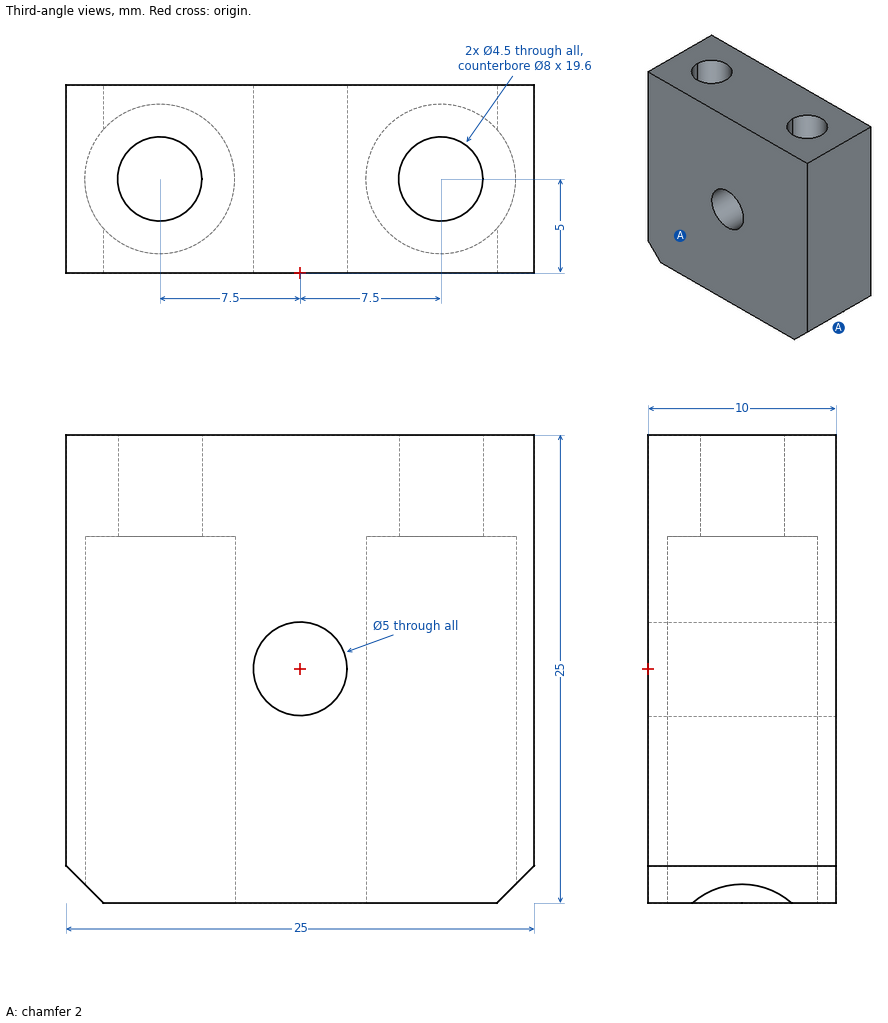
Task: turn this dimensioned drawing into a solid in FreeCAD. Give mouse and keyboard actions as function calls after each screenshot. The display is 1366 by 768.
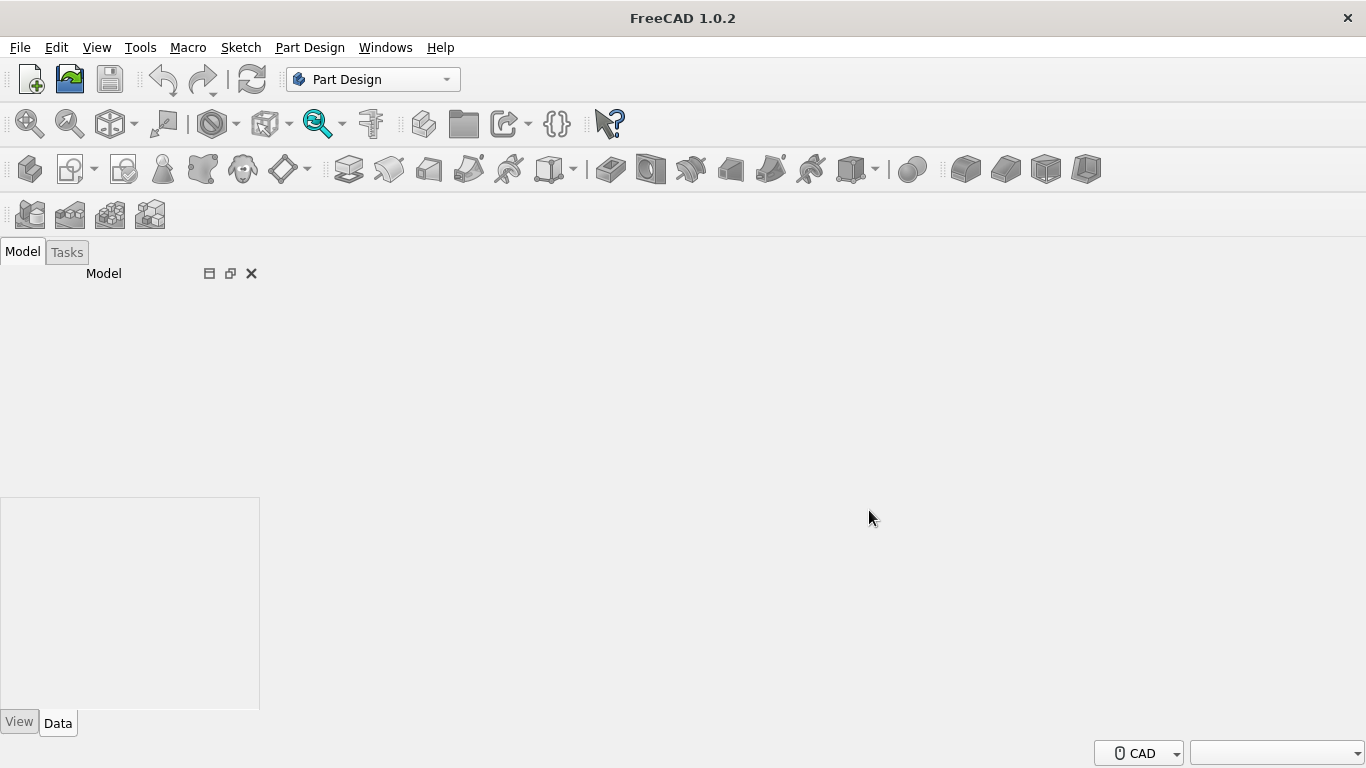
key(ctrl+n)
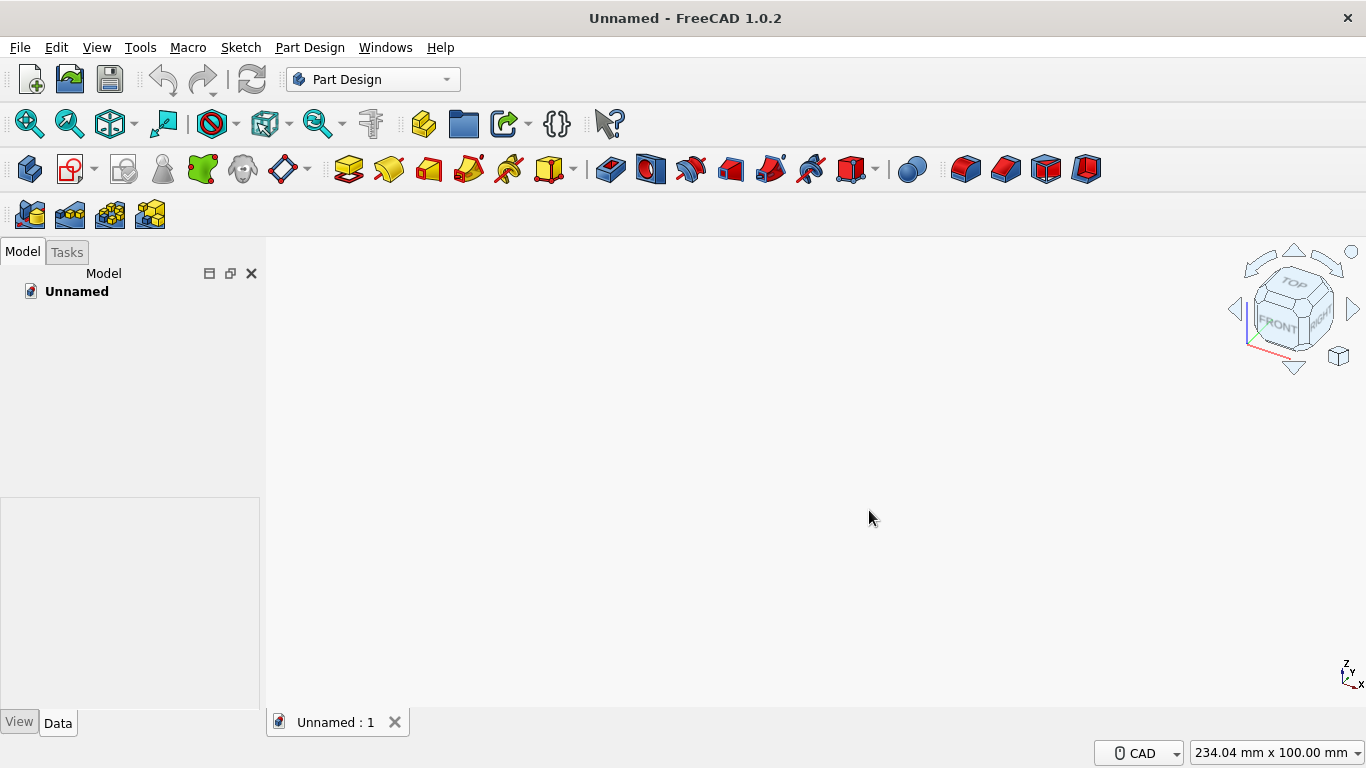
click(70, 170)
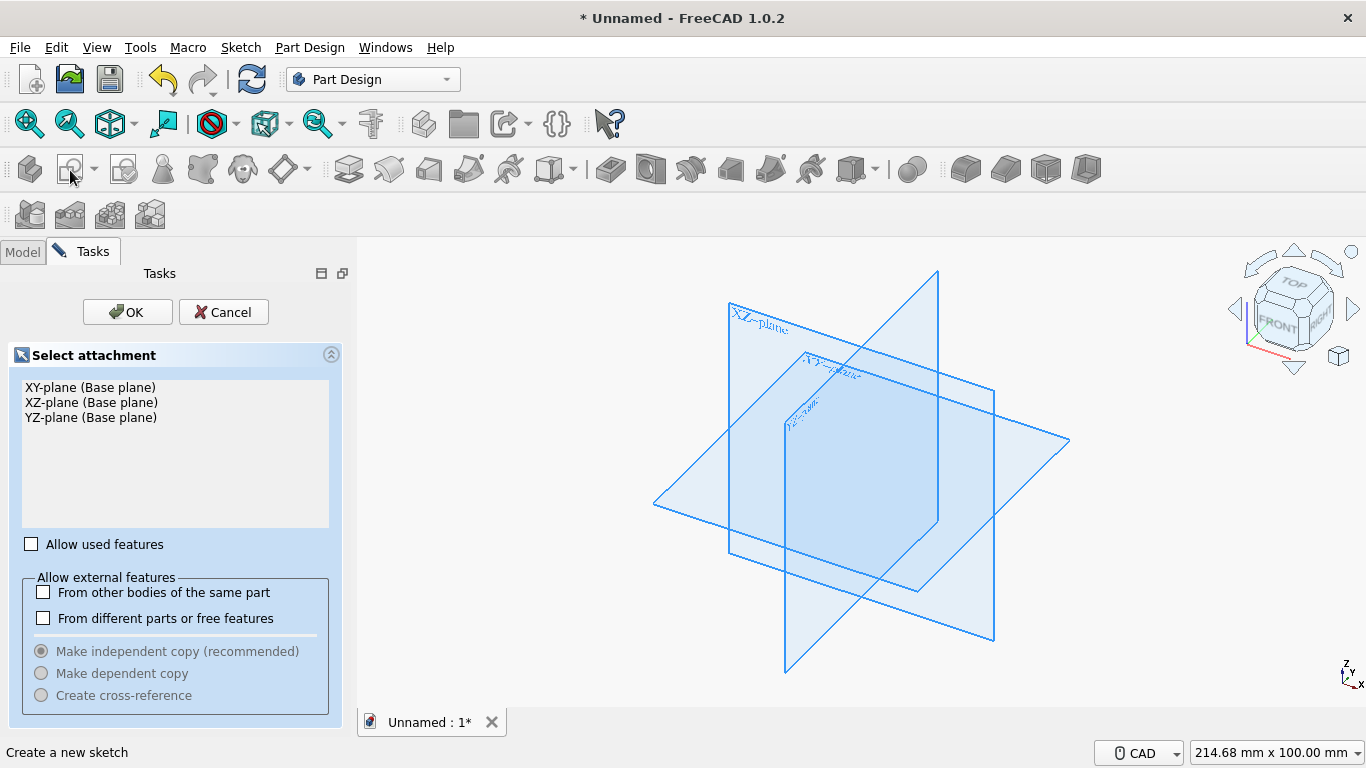
click(82, 402)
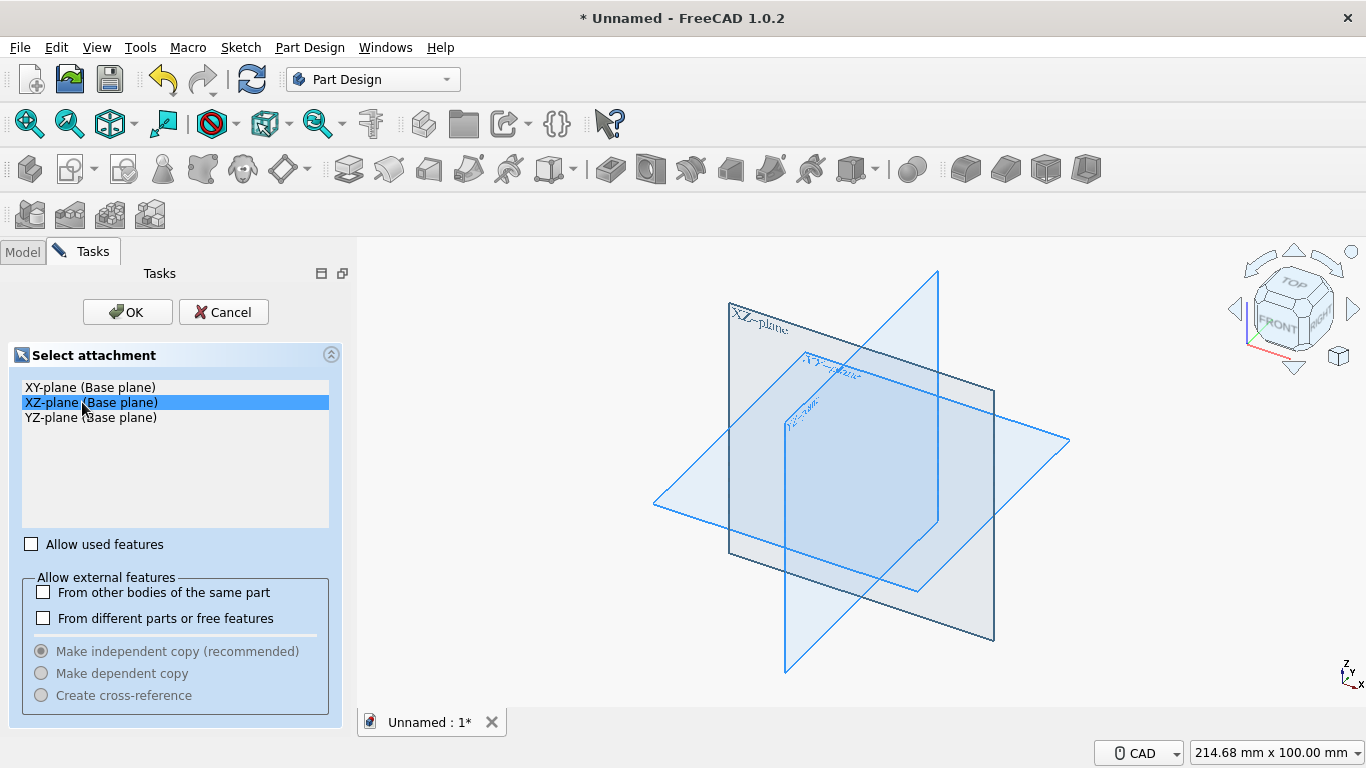
click(128, 312)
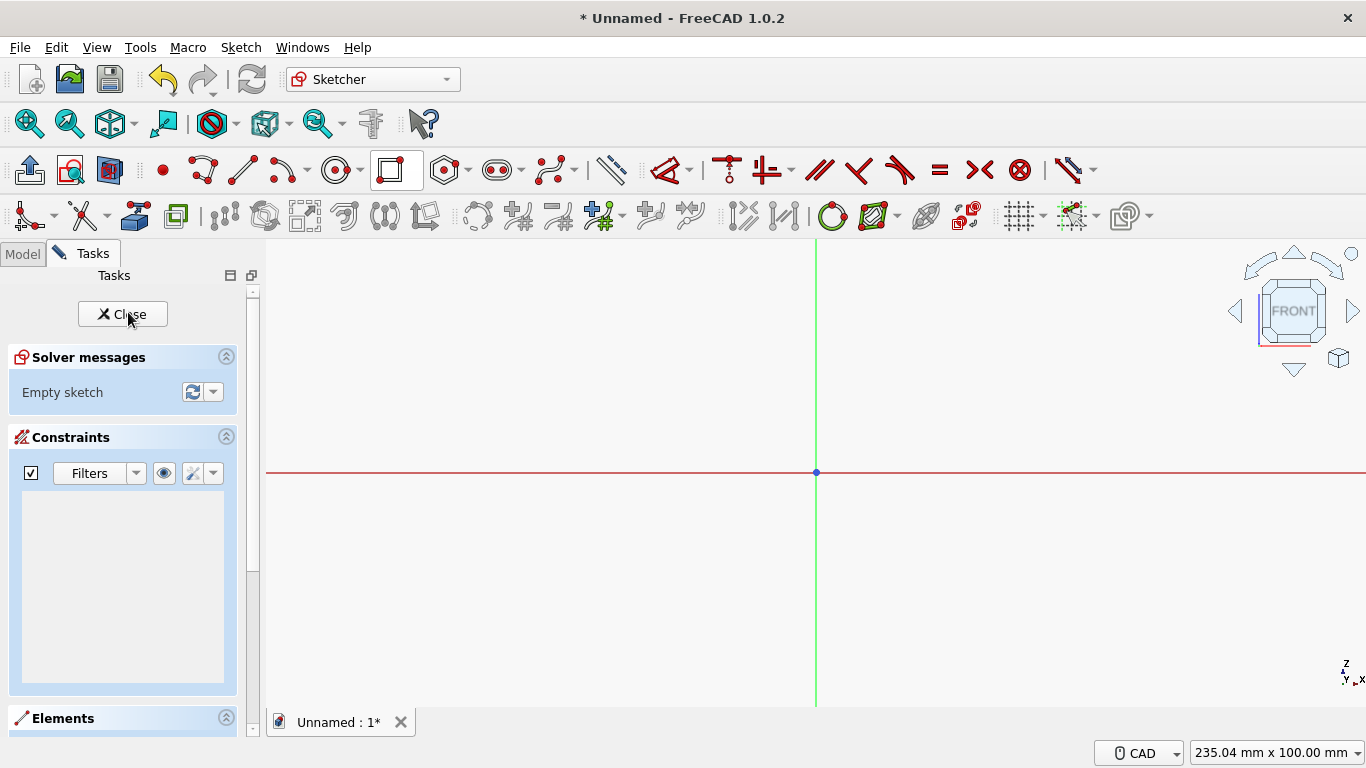
scroll(856, 473, up, 5)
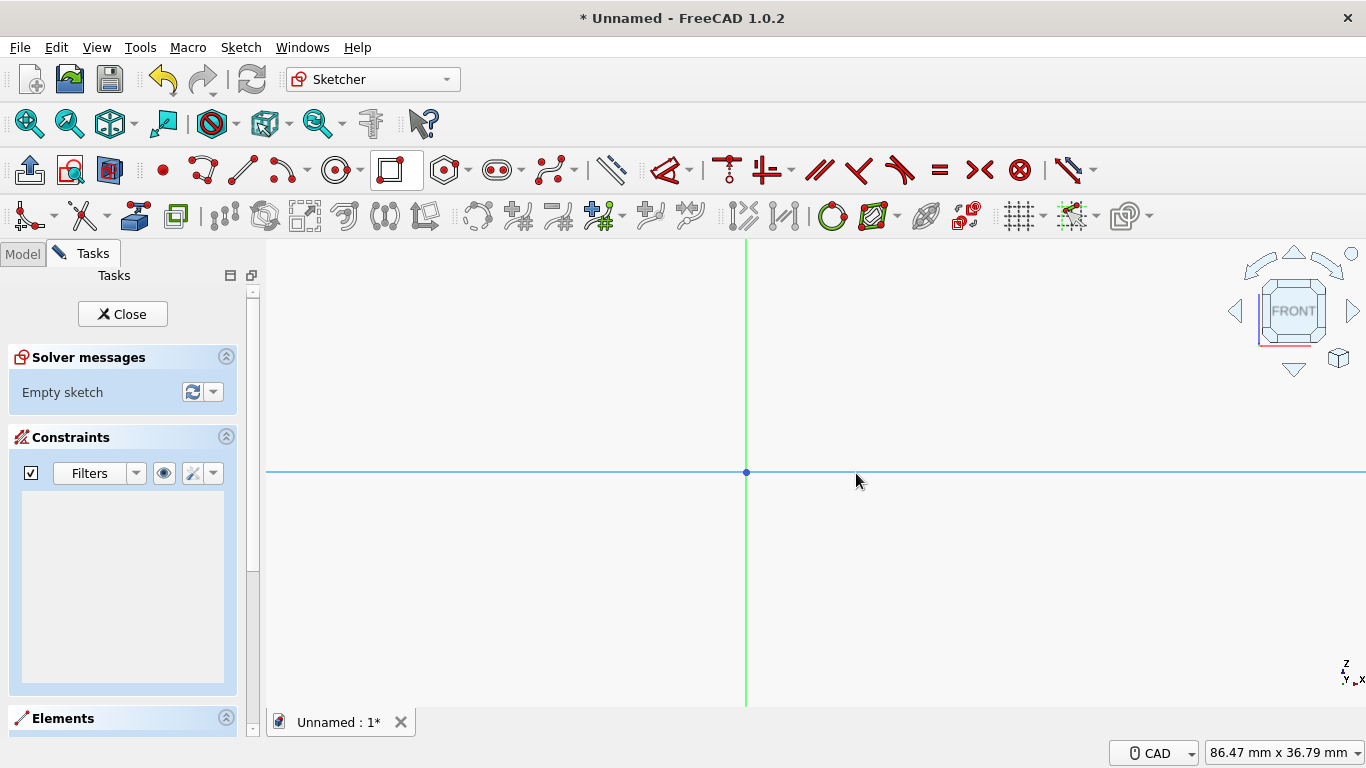
key(g)
key(v)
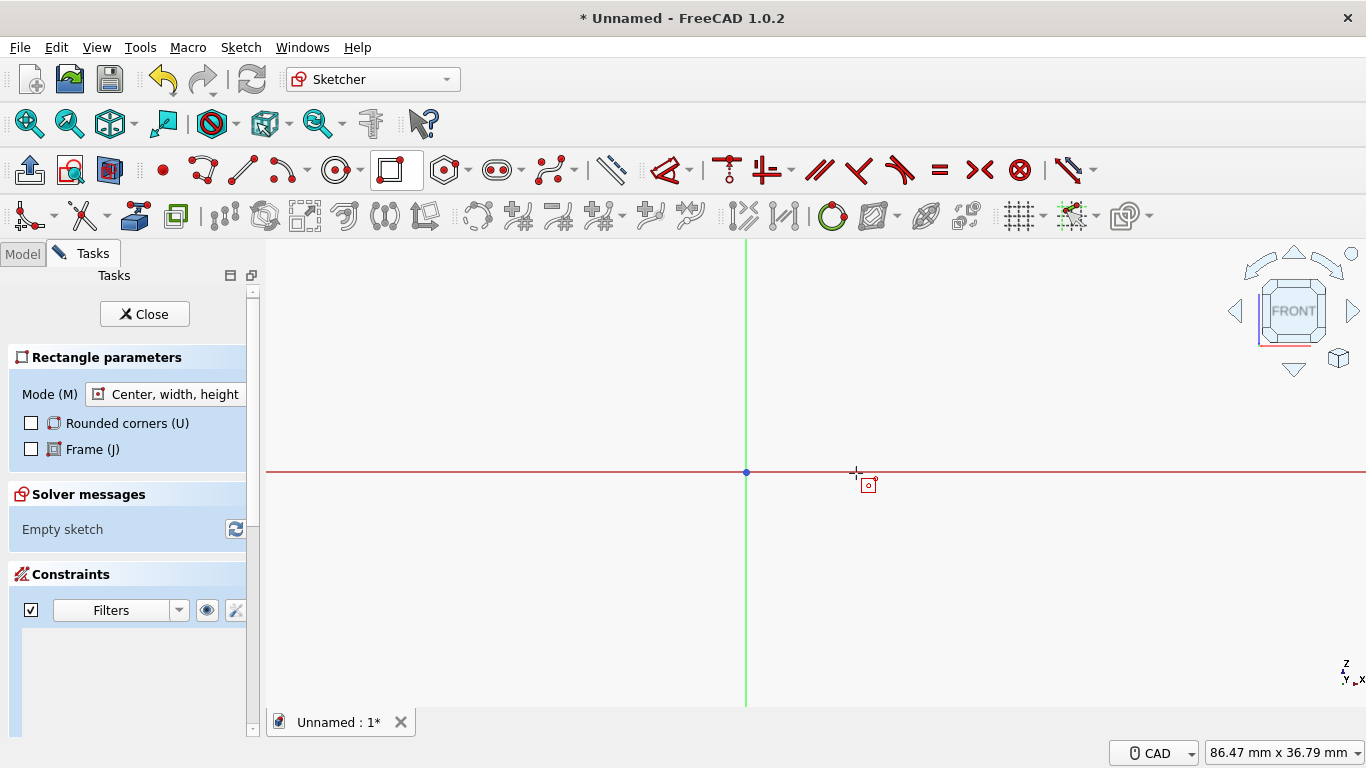
click(746, 472)
move(905, 313)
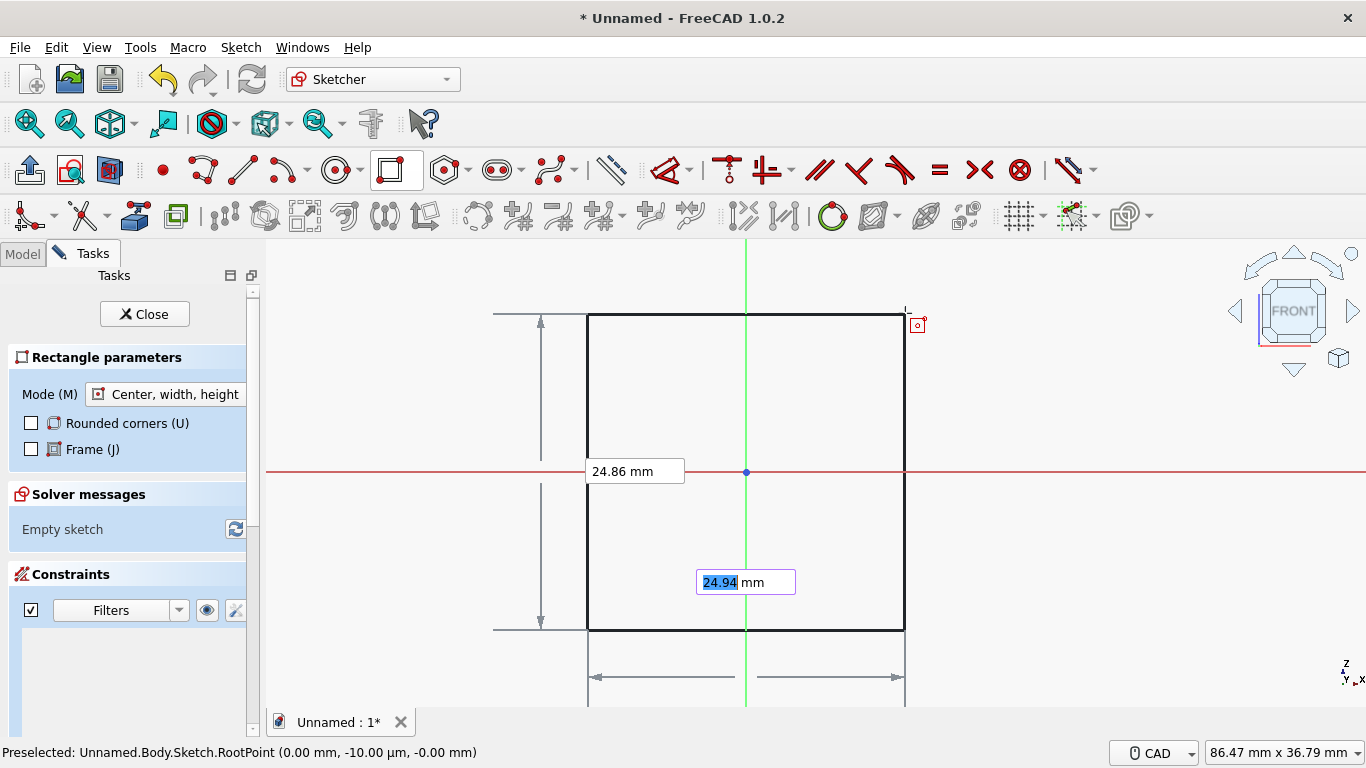
text(25)
key(Tab)
text(25)
key(Return)
key(Escape)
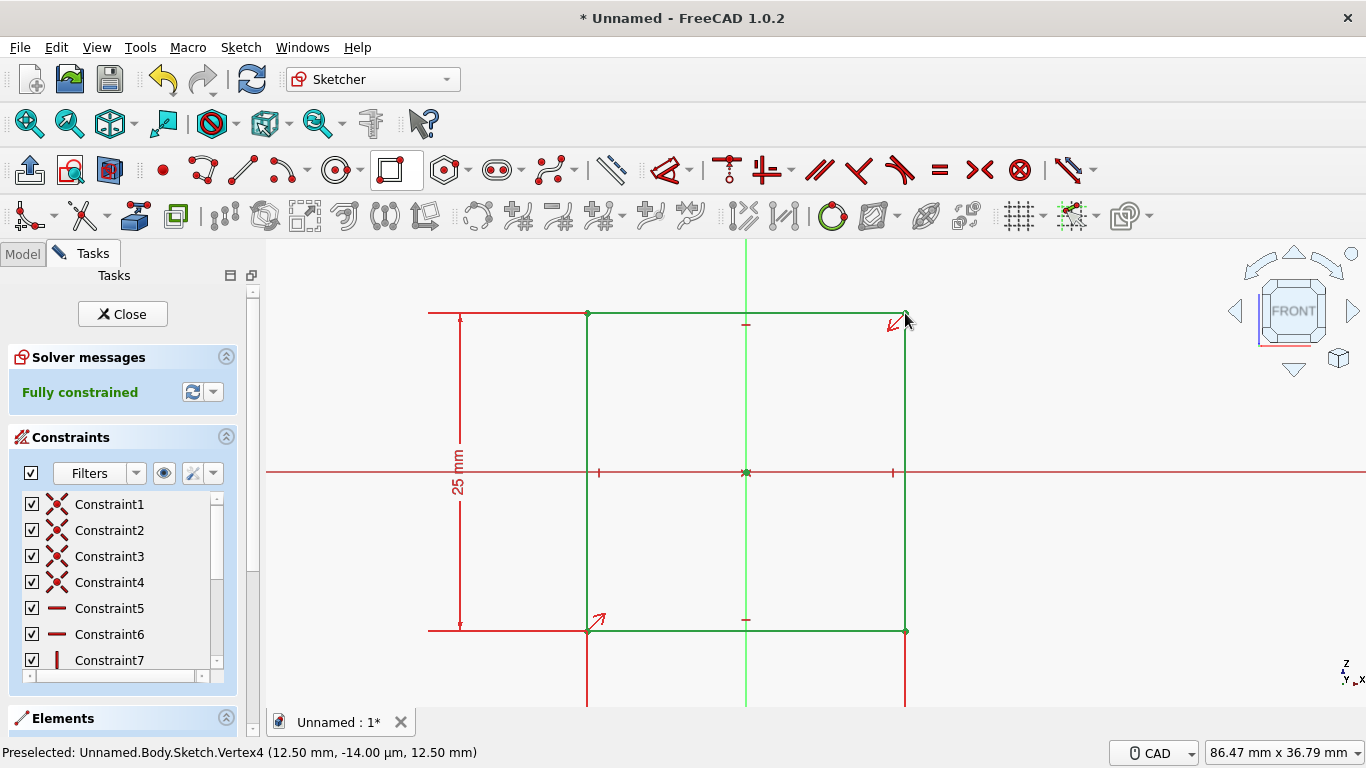
click(123, 314)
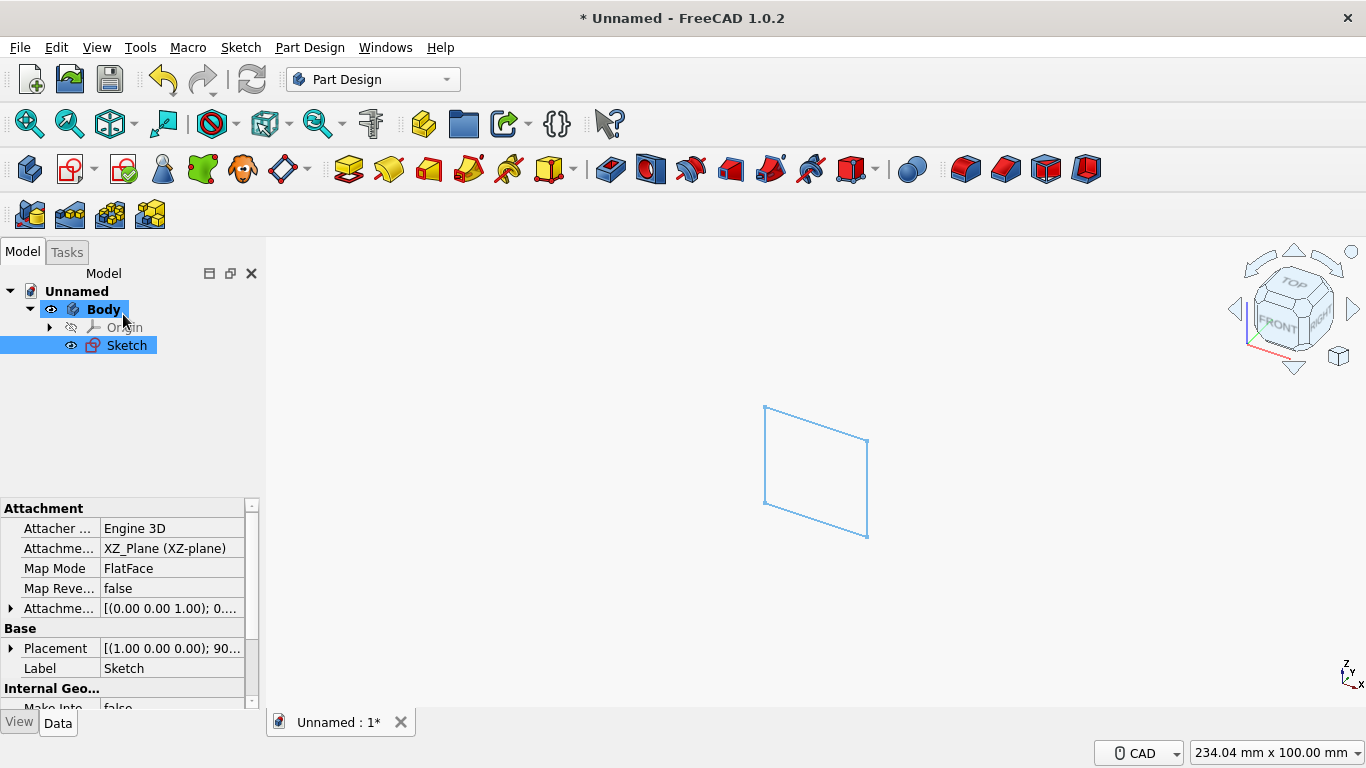
click(350, 170)